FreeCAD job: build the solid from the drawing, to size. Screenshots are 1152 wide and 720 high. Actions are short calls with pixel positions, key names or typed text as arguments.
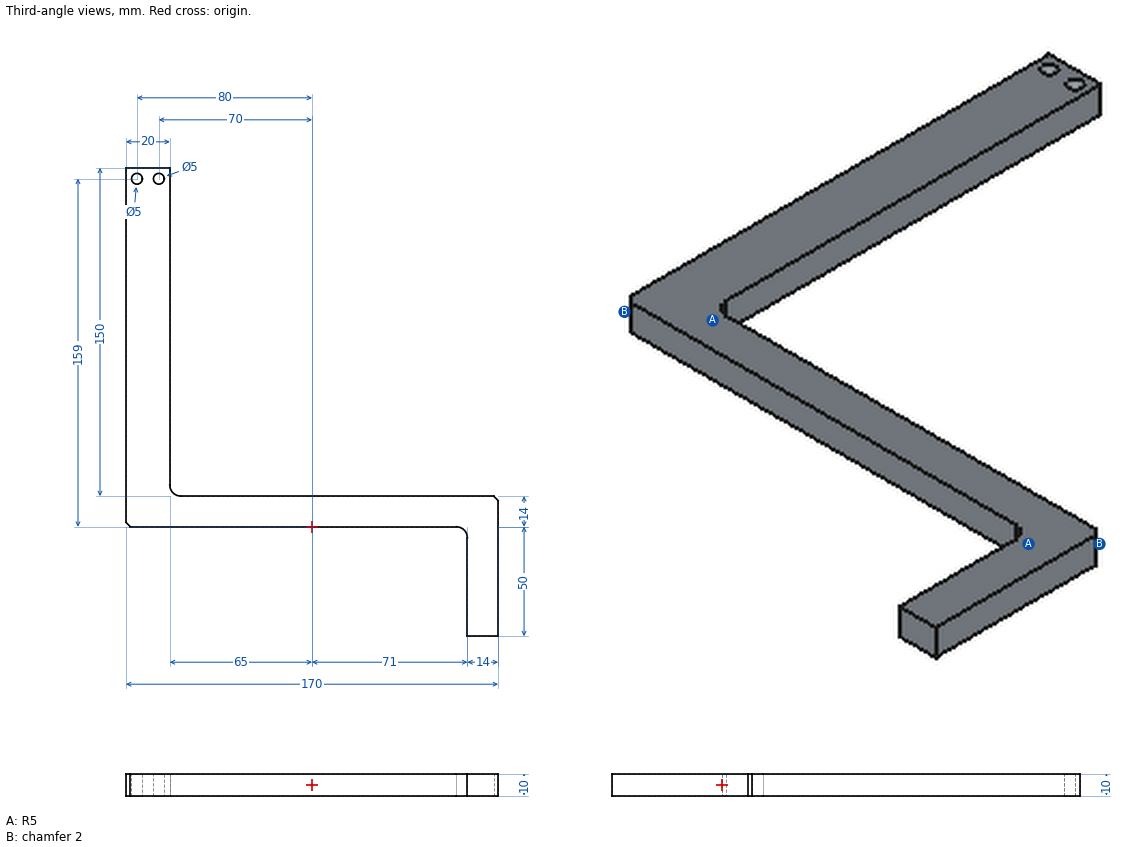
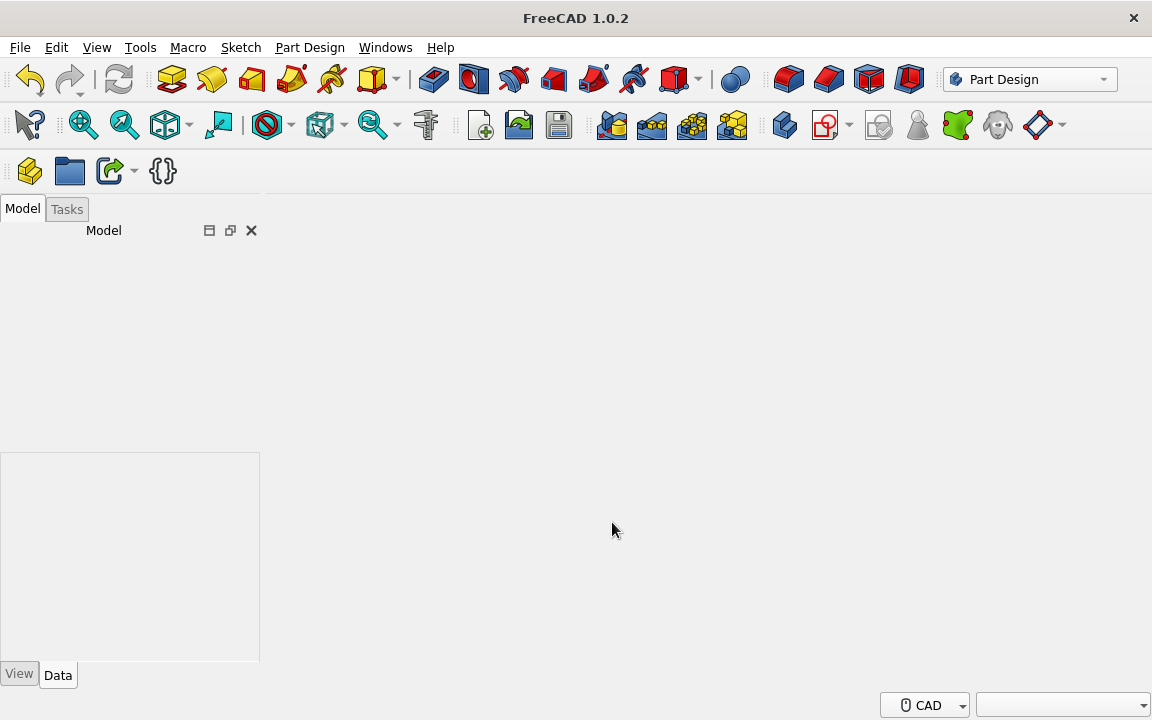
key(ctrl+n)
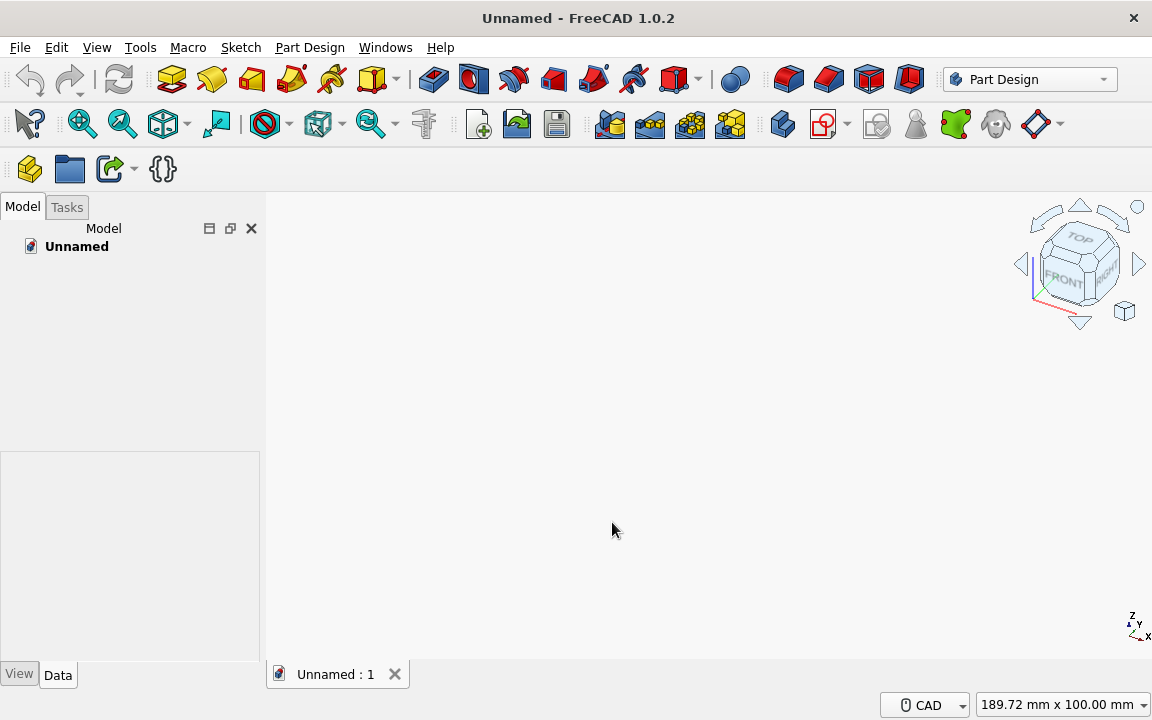
click(824, 124)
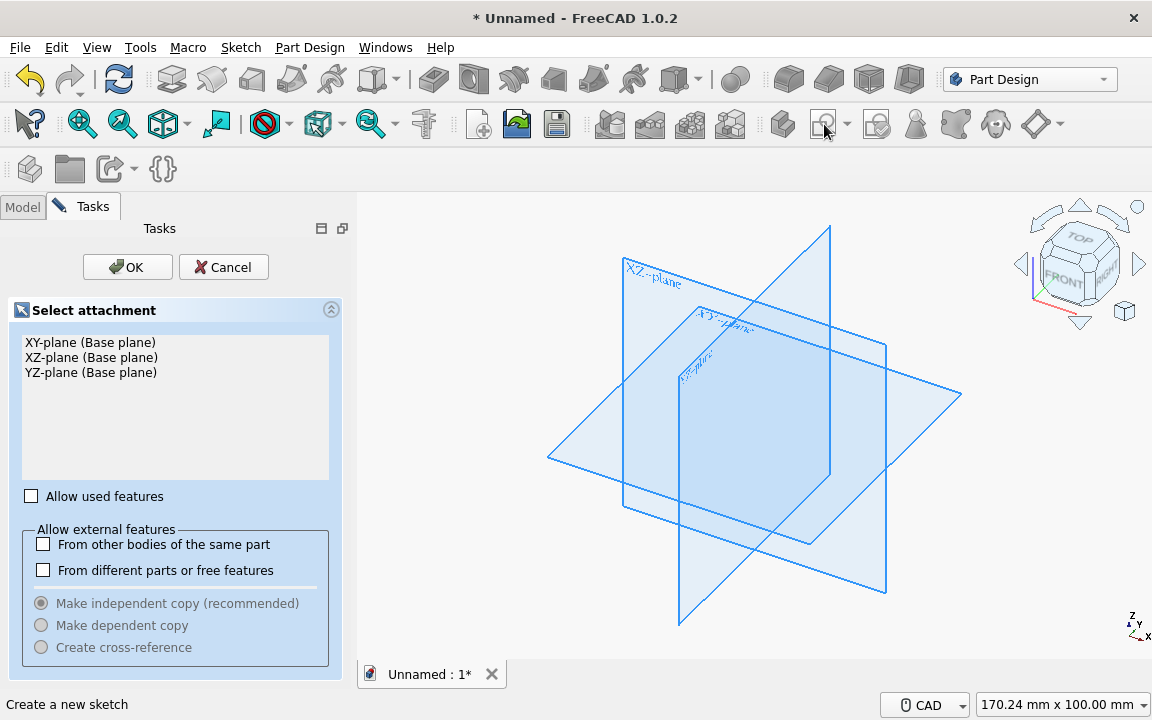
click(82, 342)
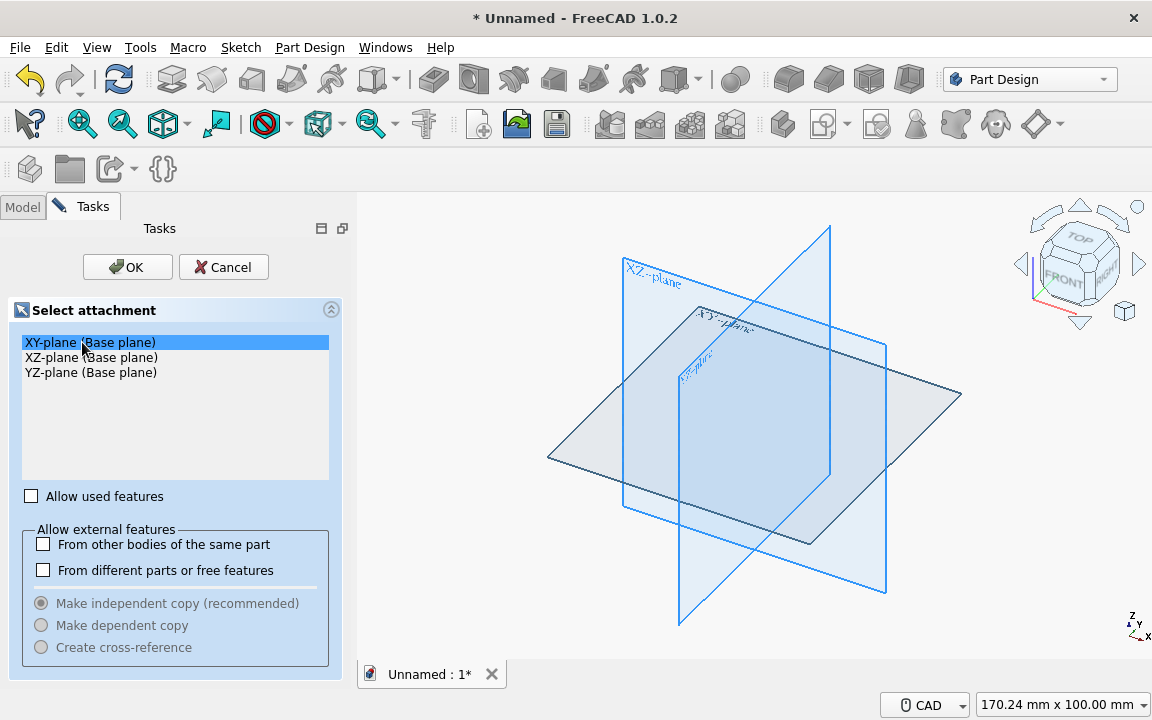
click(128, 267)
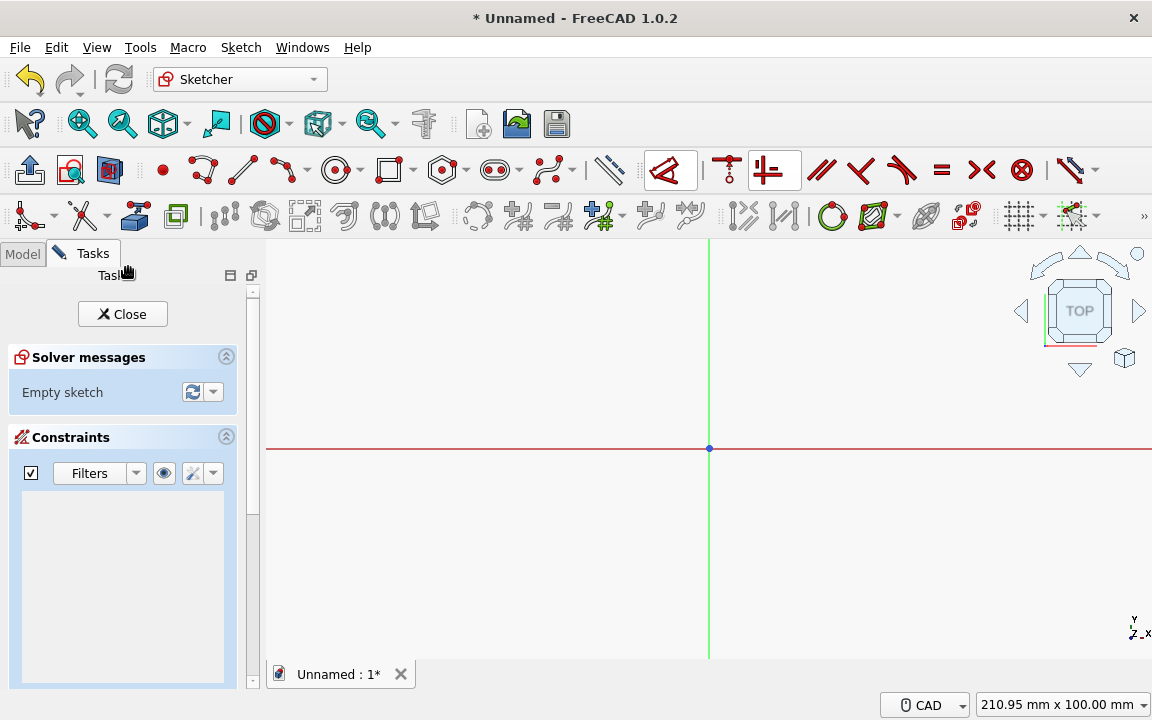
scroll(601, 631, down, 5)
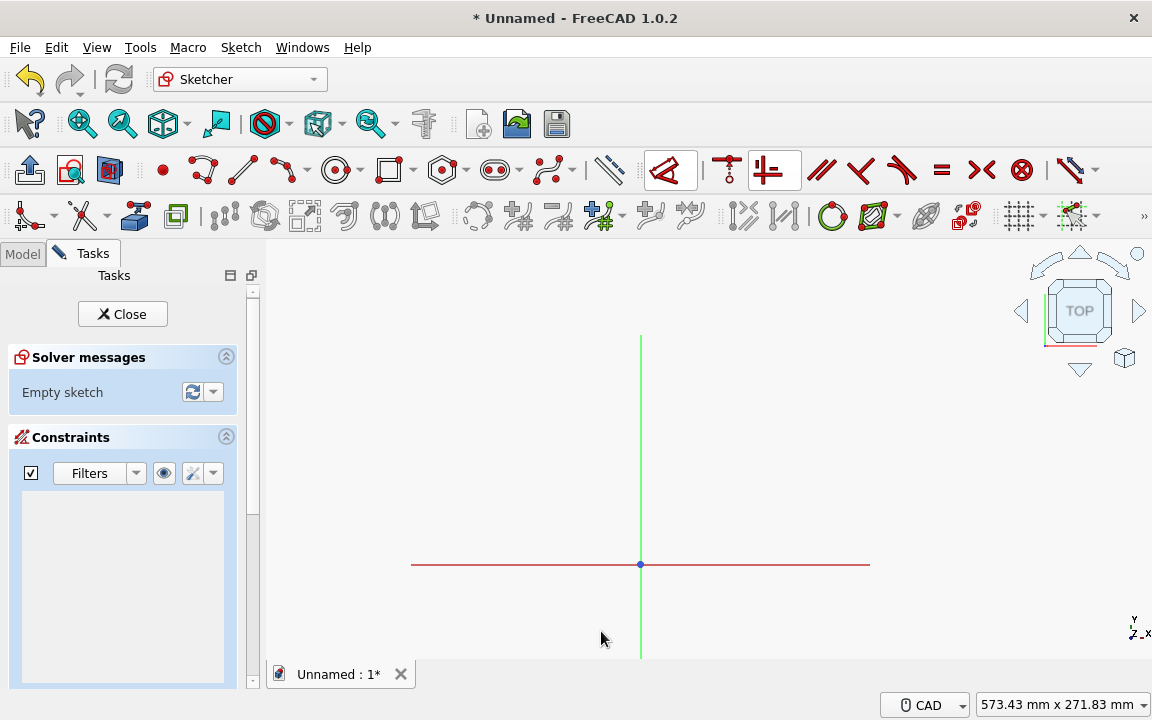
click(204, 170)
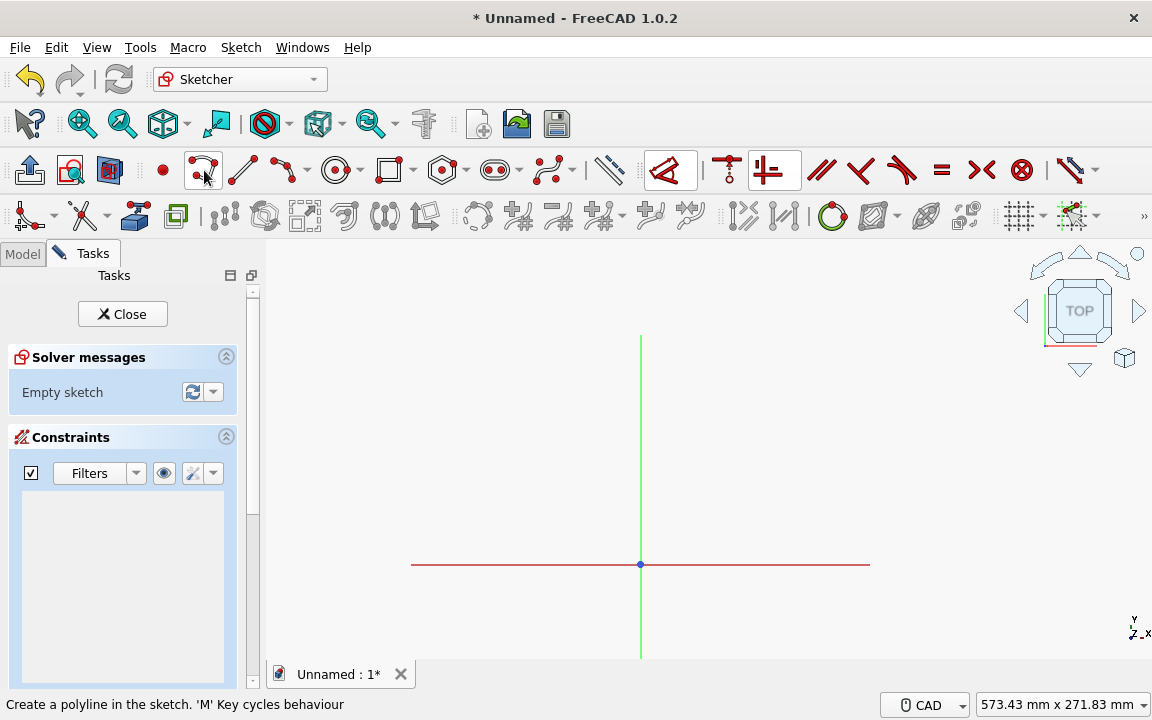
click(541, 543)
click(541, 311)
click(510, 311)
click(510, 565)
click(772, 556)
click(772, 543)
click(541, 544)
key(Escape)
key(Escape)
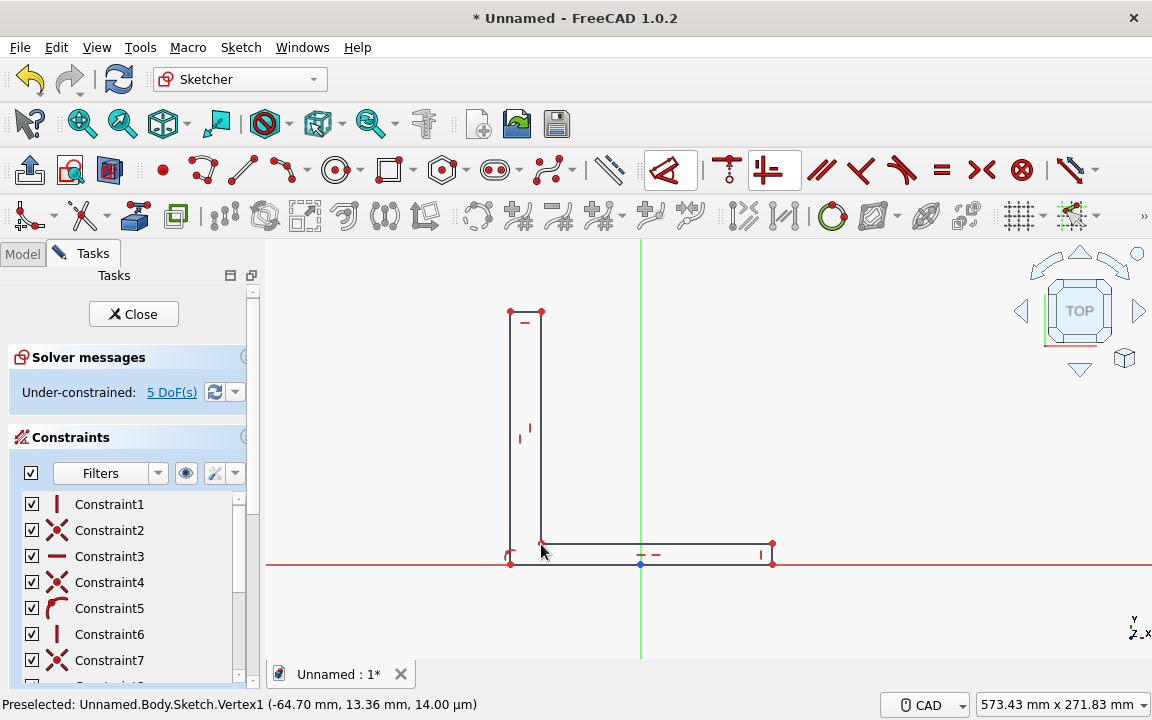
key(d)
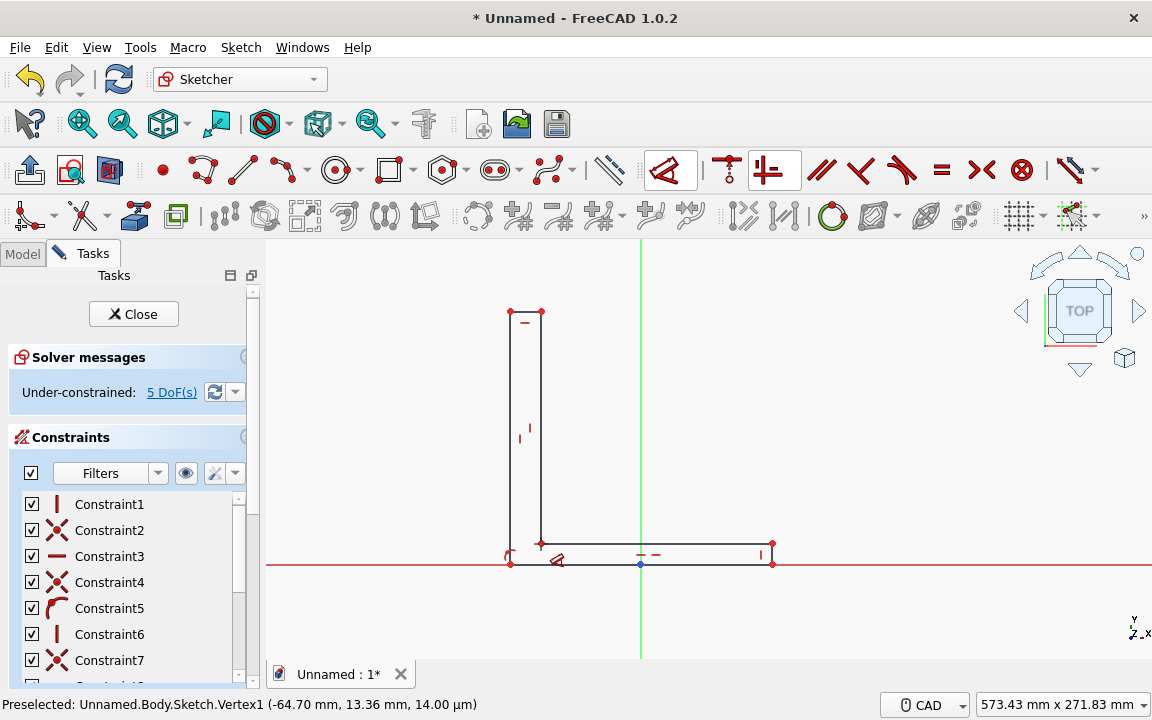
scroll(532, 312, up, 2)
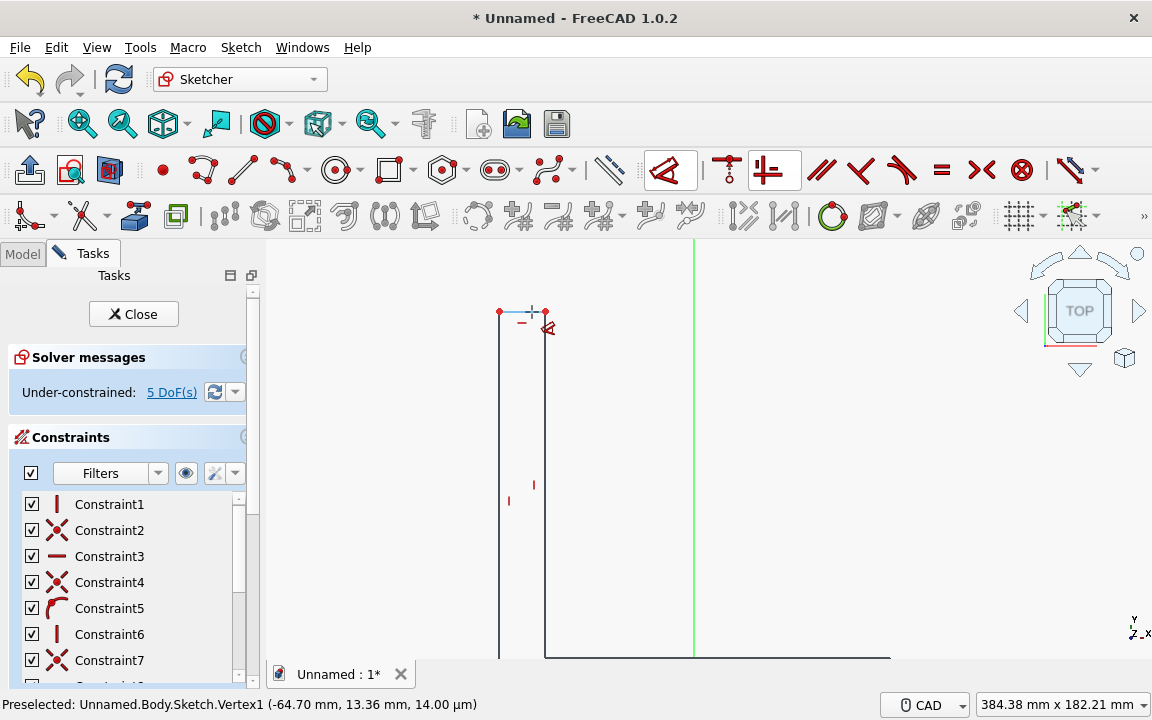
click(531, 312)
click(522, 278)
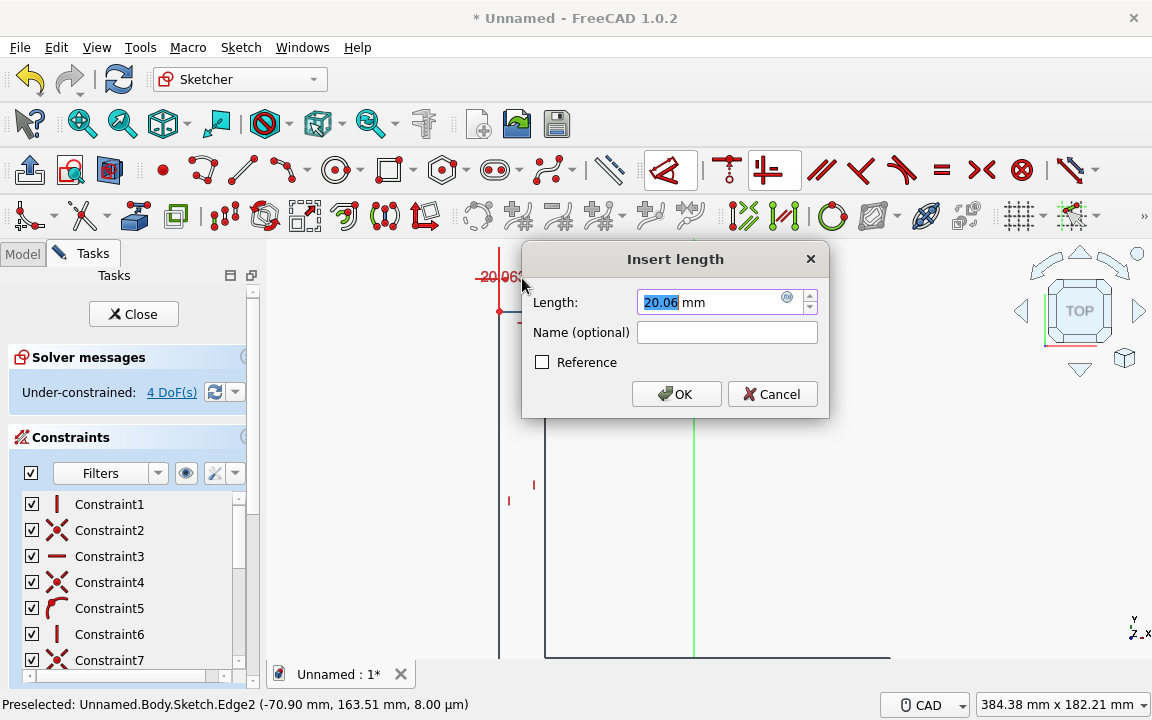
text(20)
key(Return)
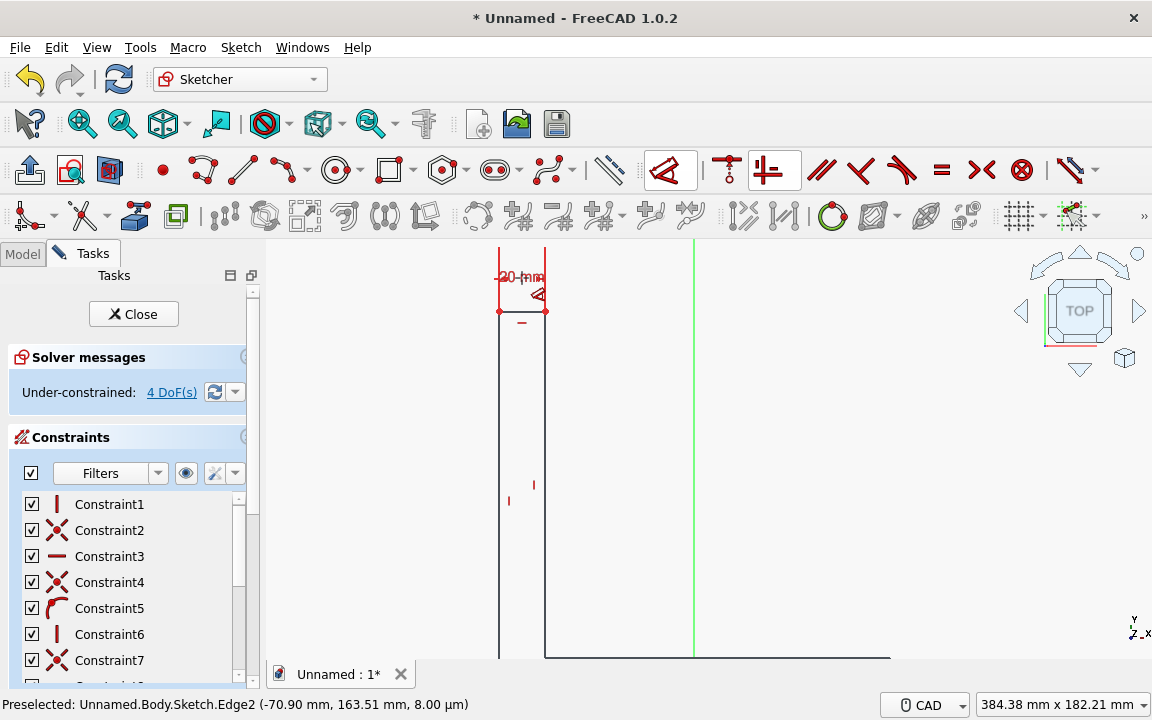
scroll(531, 346, down, 2)